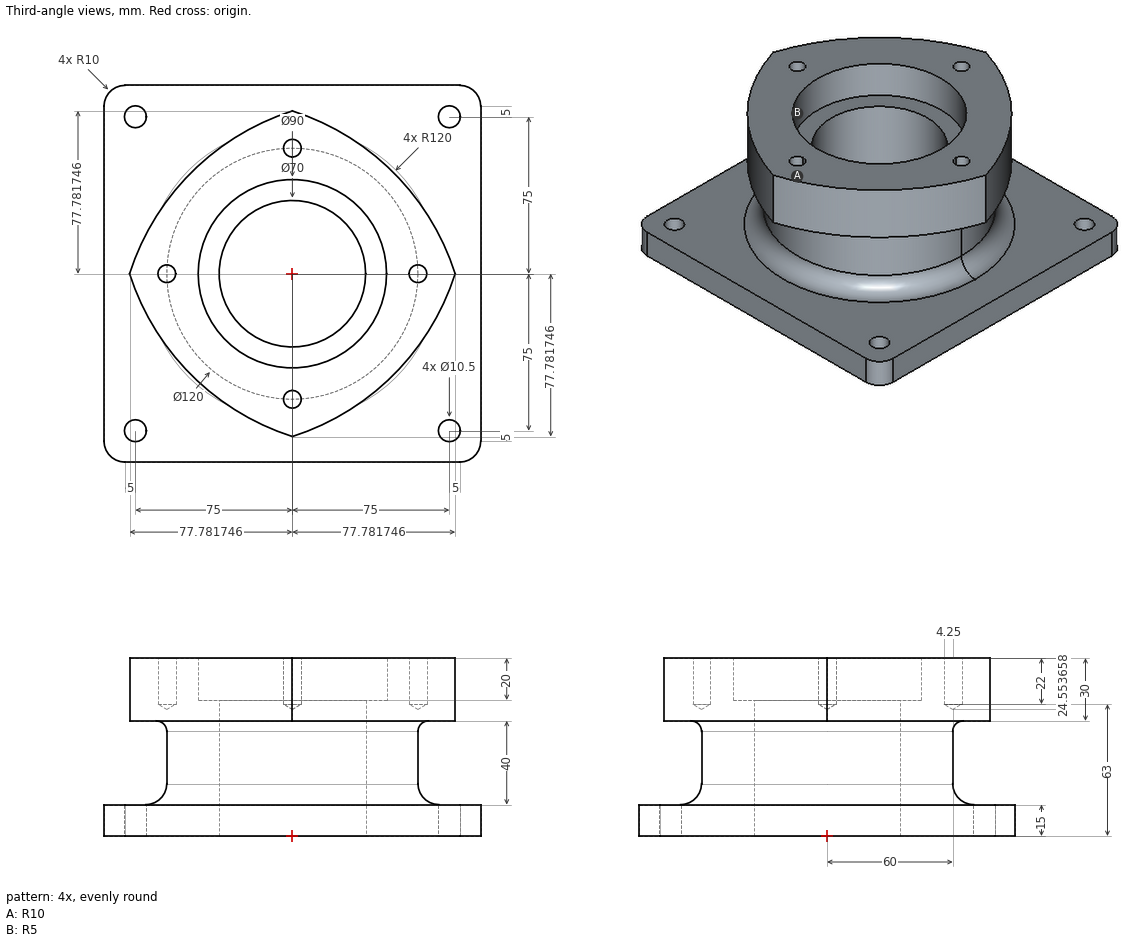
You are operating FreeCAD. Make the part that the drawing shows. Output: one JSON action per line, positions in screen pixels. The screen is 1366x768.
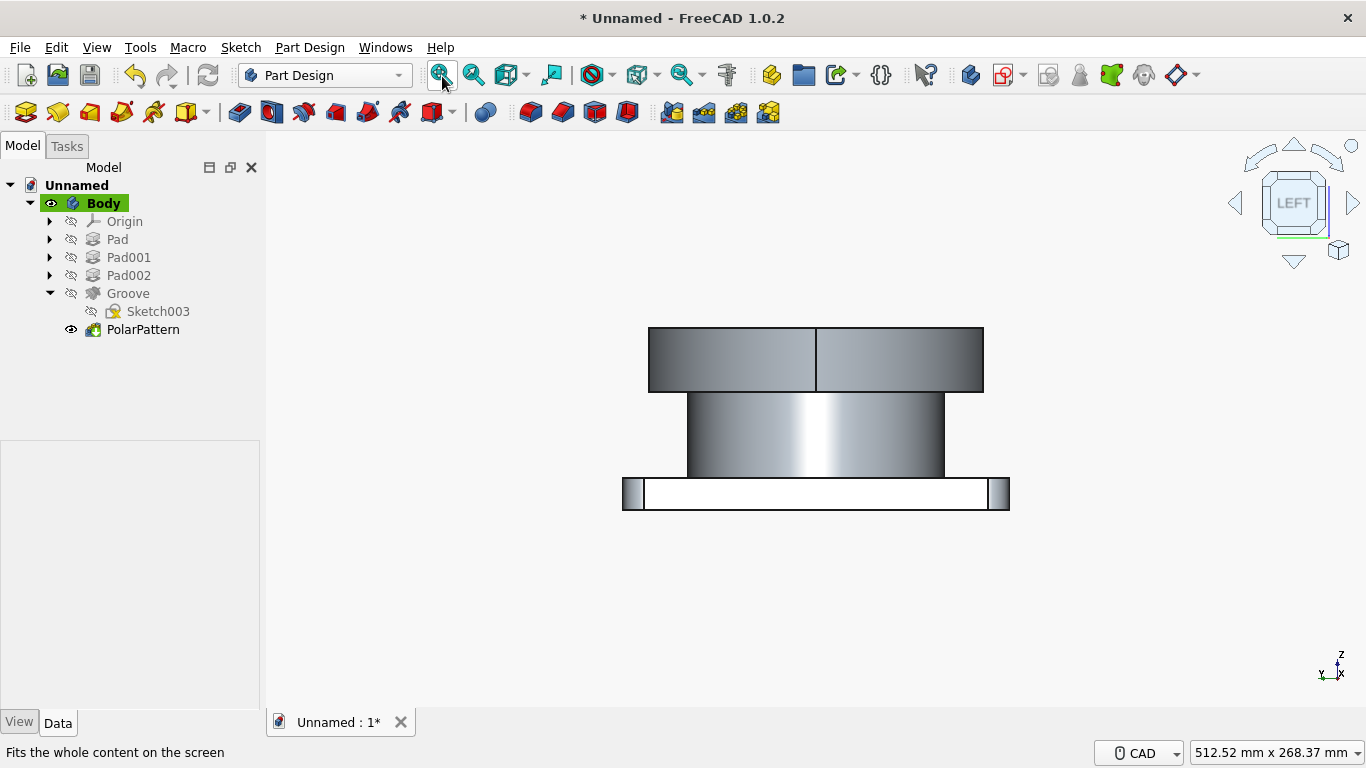
{"action": "left_click", "coordinate": [442, 76]}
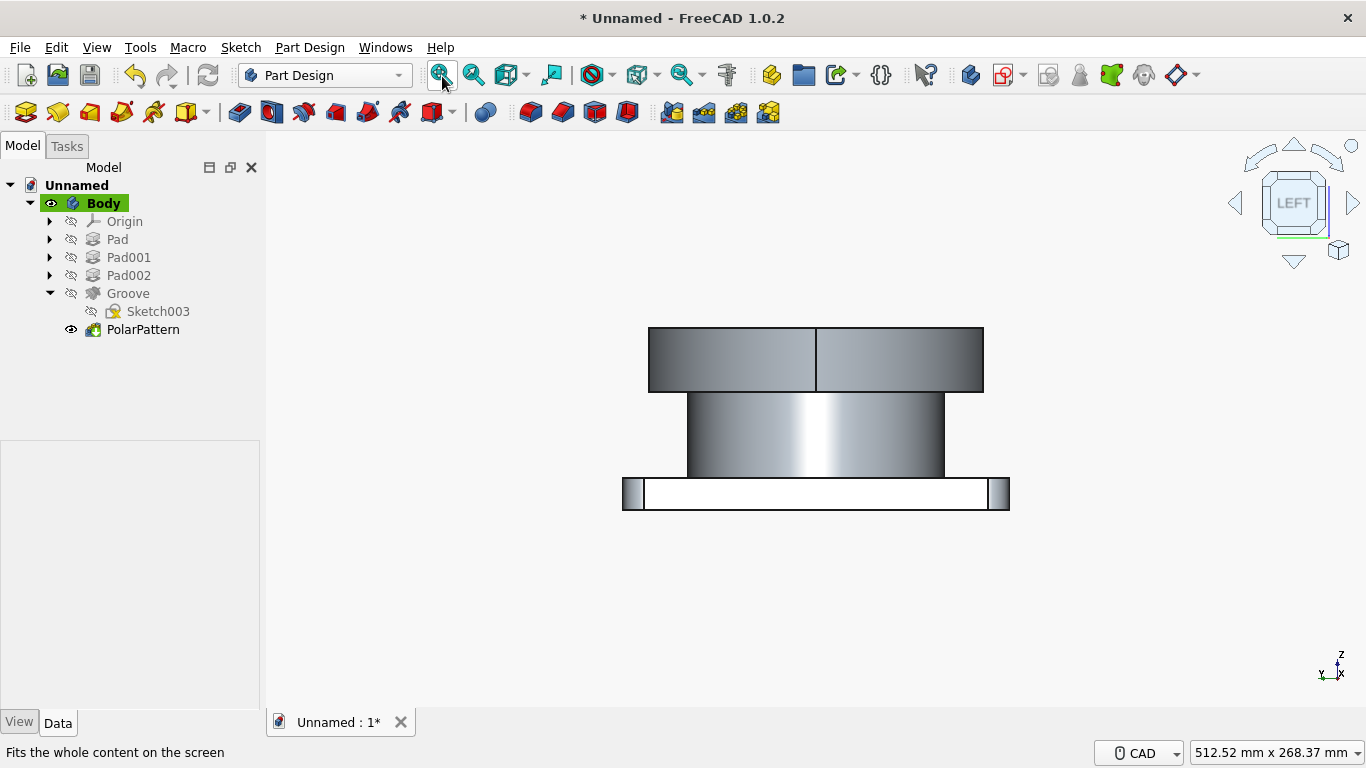
{"action": "key", "text": "v 3"}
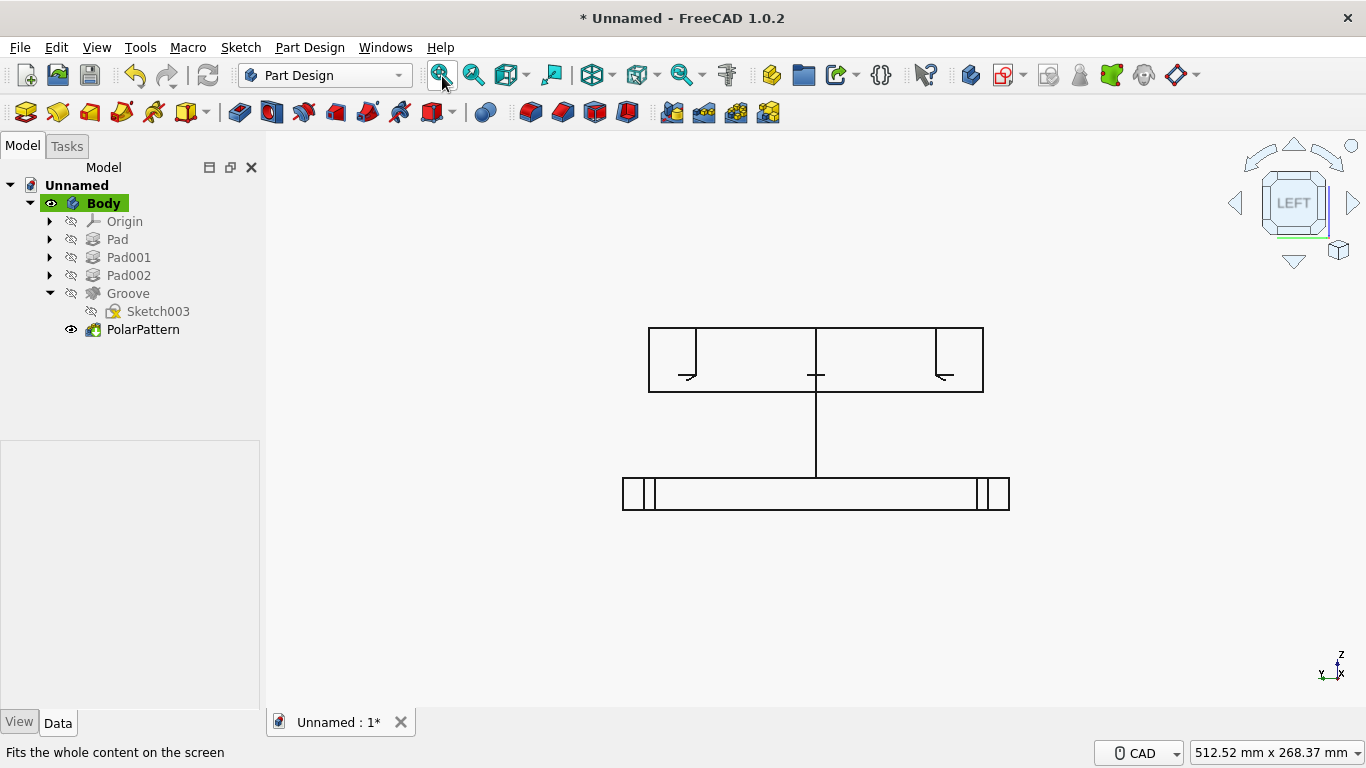
{"action": "key", "text": "0"}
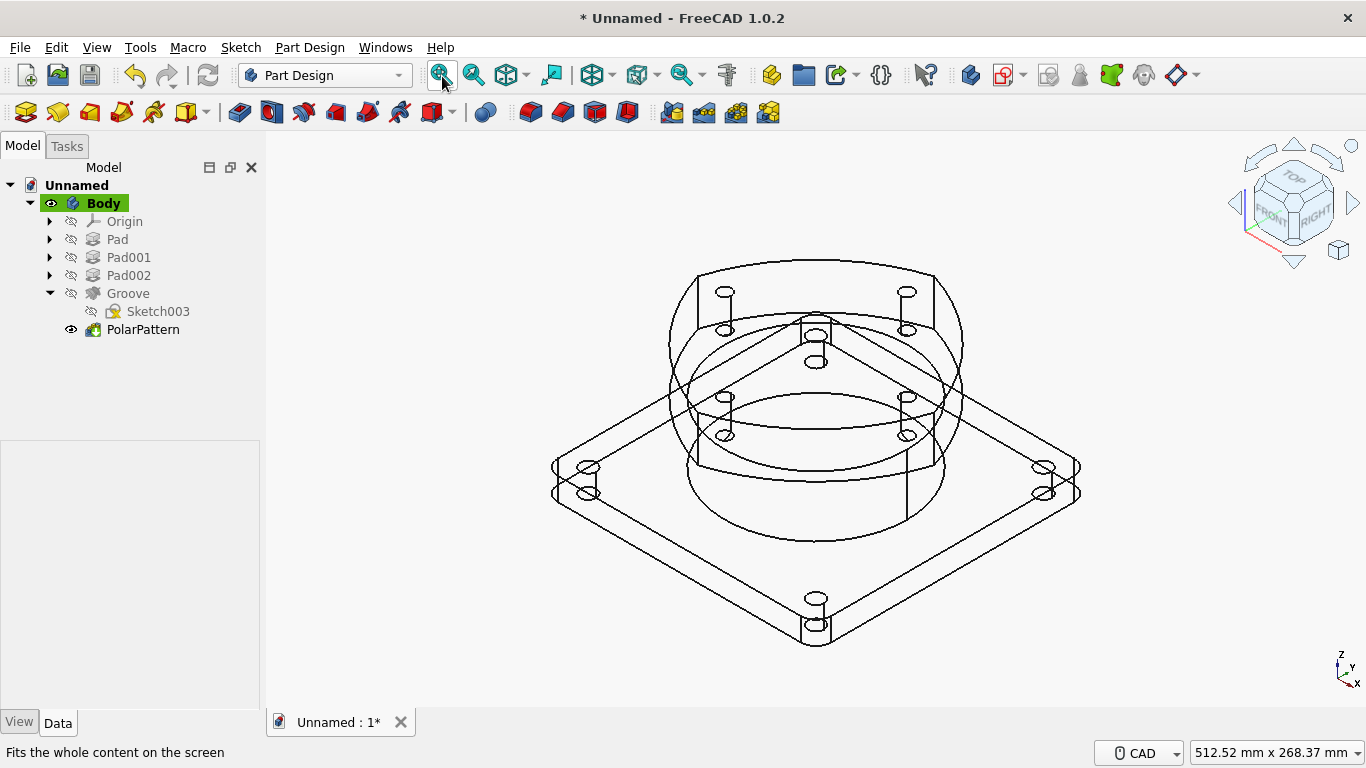
{"action": "left_click", "coordinate": [796, 393]}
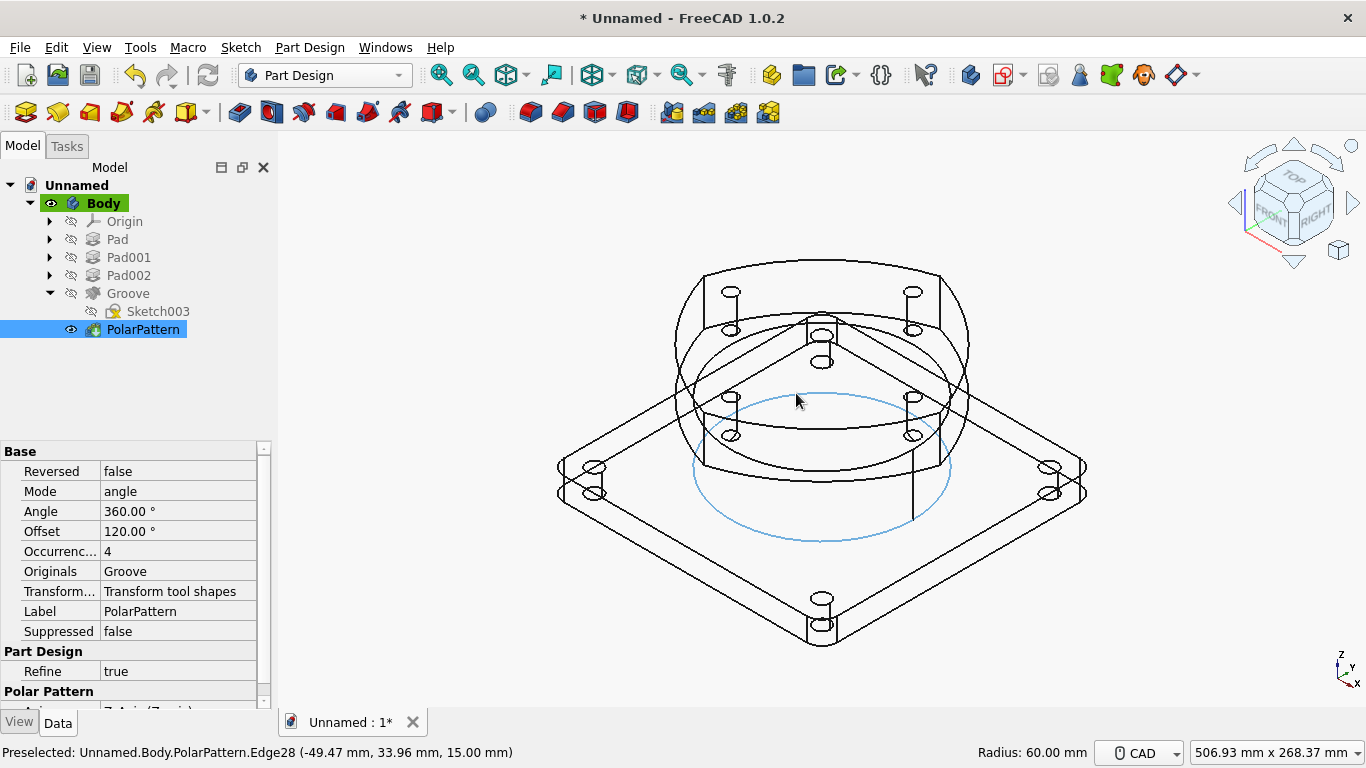
{"action": "key", "text": "v 1"}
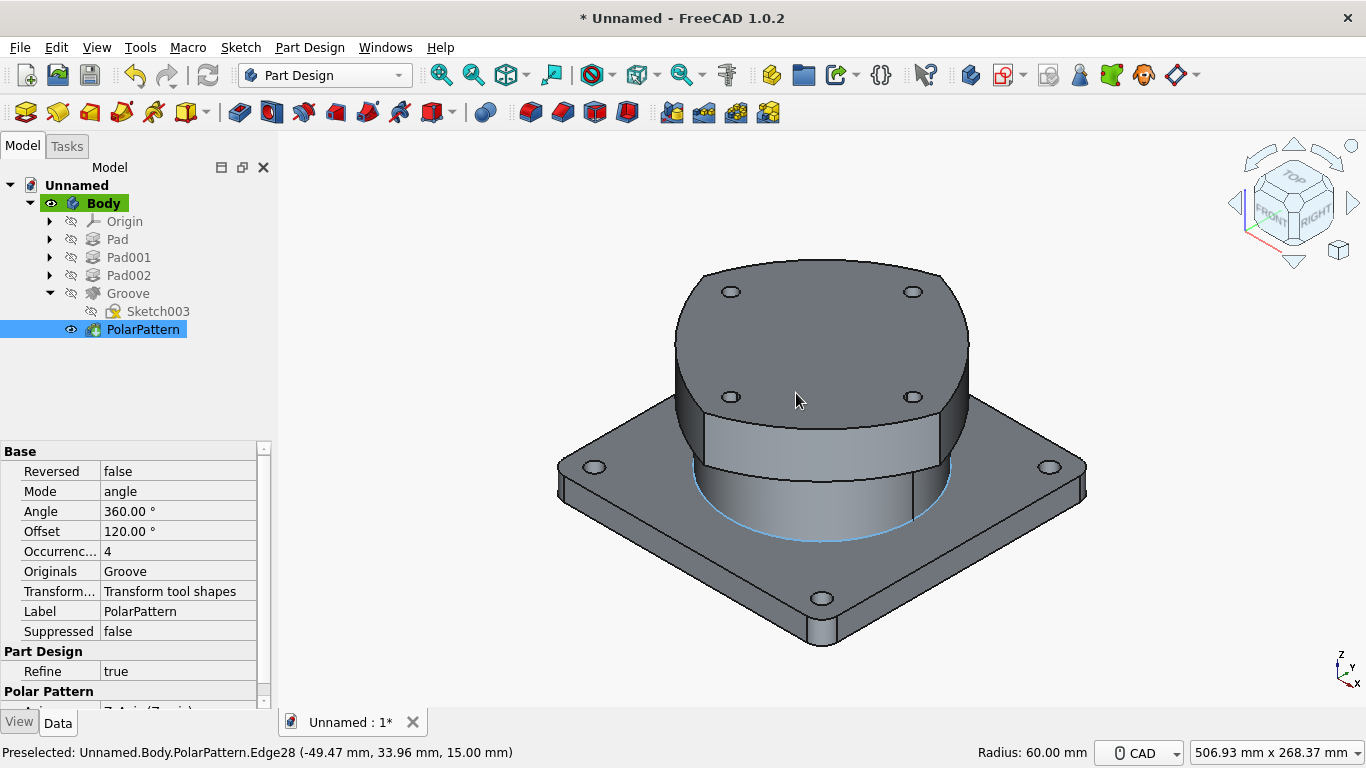
{"action": "left_click", "coordinate": [532, 112]}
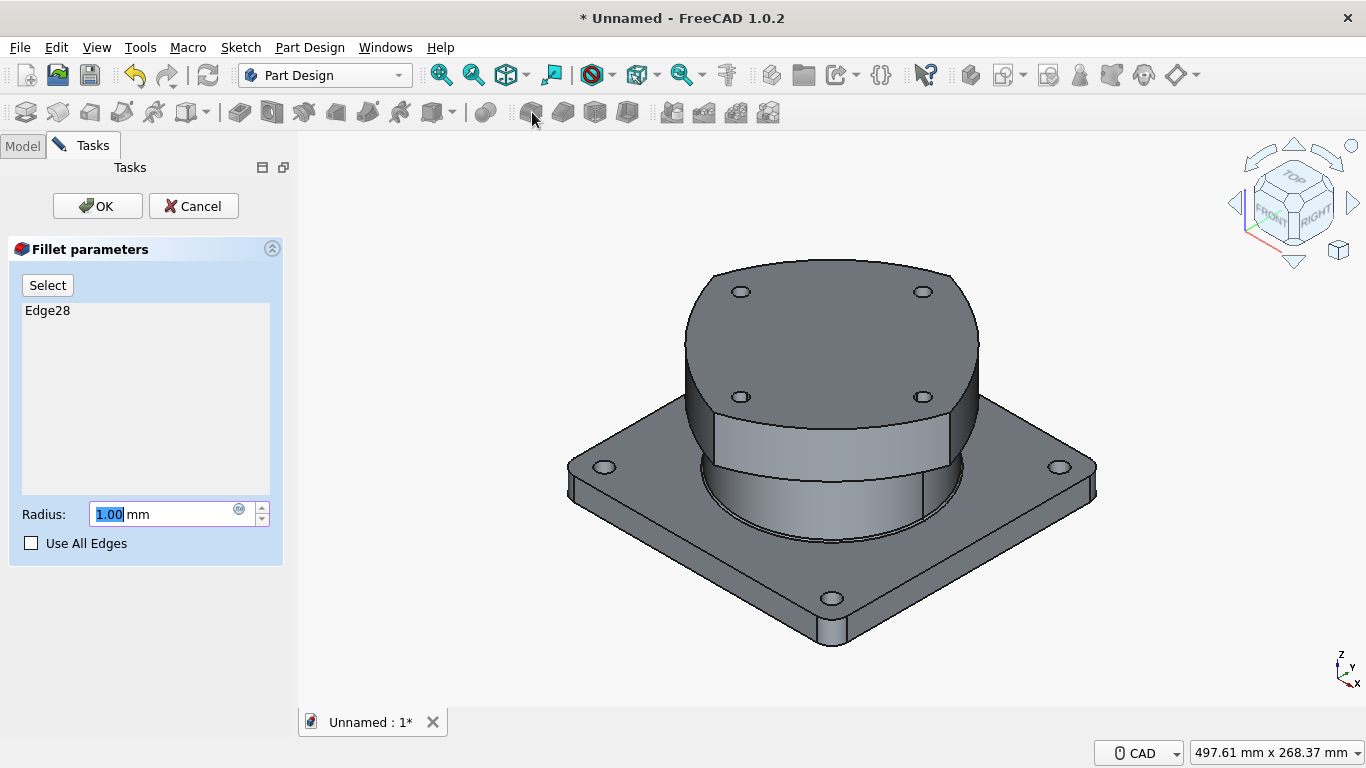
{"action": "type", "text": "10"}
{"action": "key", "text": "Tab"}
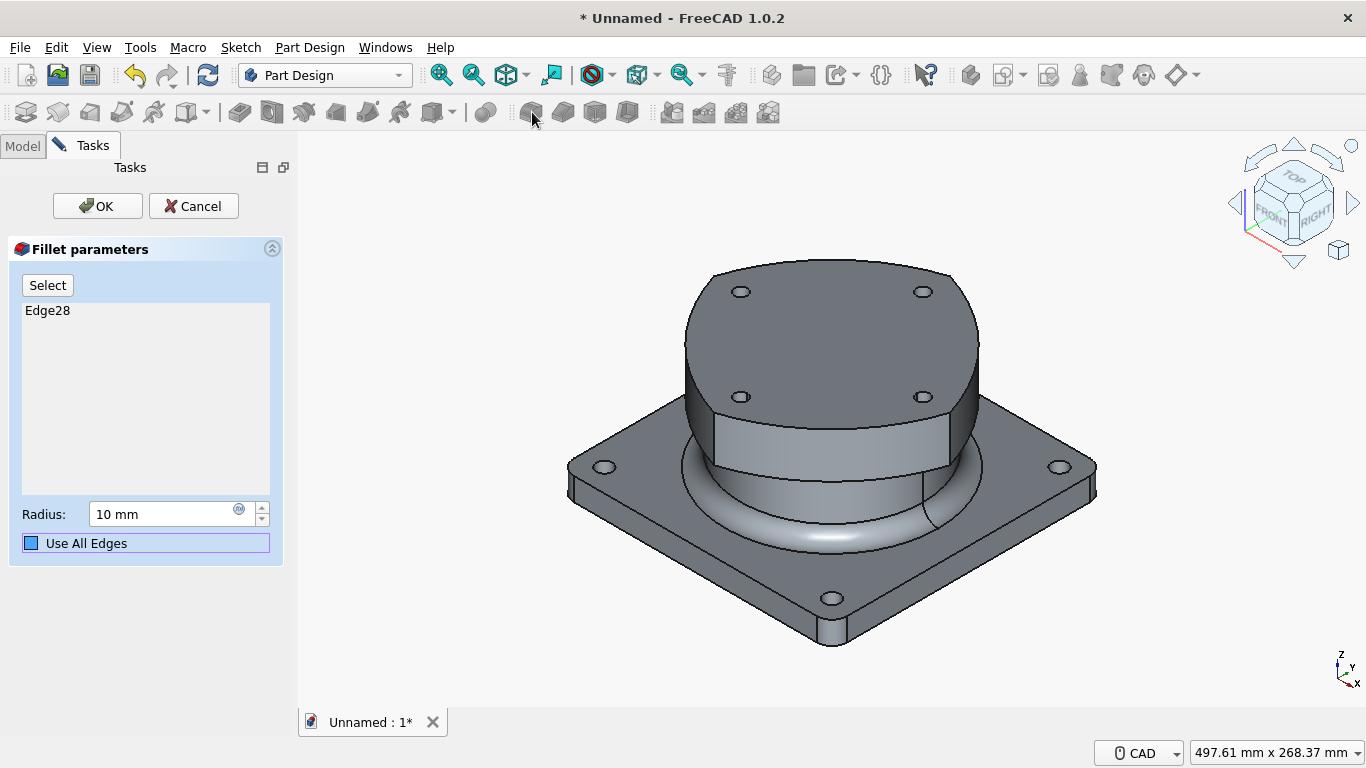
{"action": "left_click", "coordinate": [98, 206]}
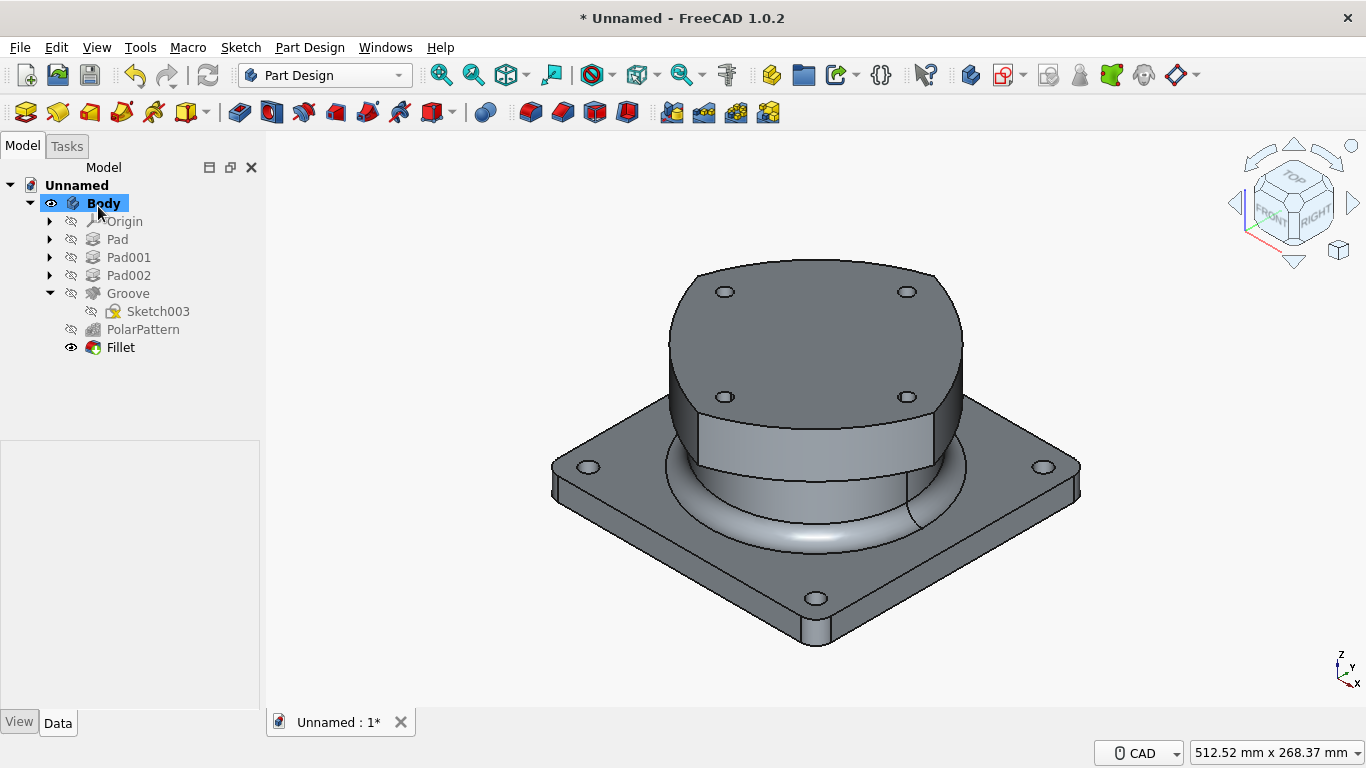
{"action": "key", "text": "2"}